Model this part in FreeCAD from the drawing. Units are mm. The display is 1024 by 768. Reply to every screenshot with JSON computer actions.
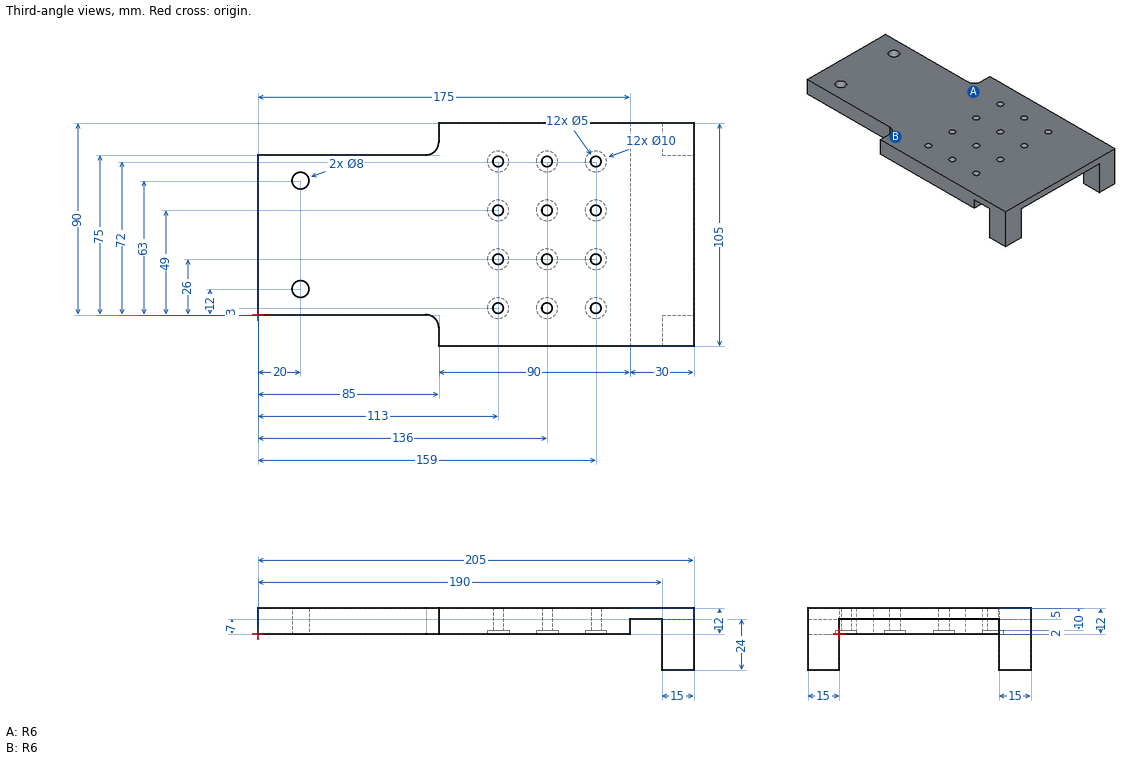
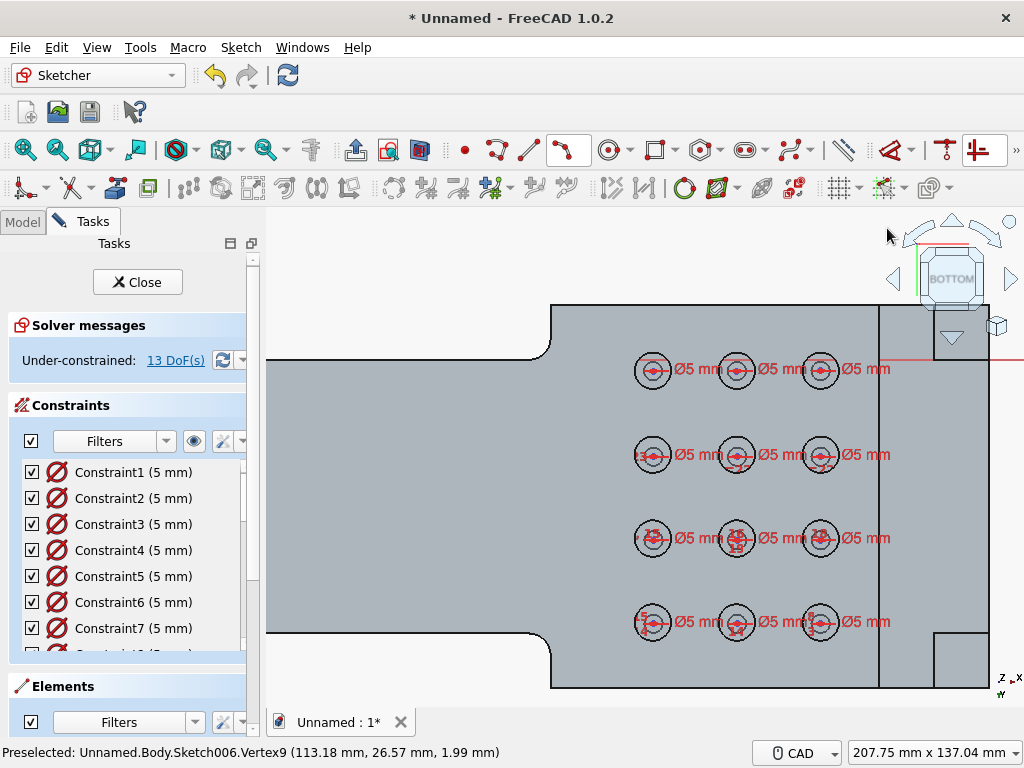
{"action": "left_click", "coordinate": [737, 457]}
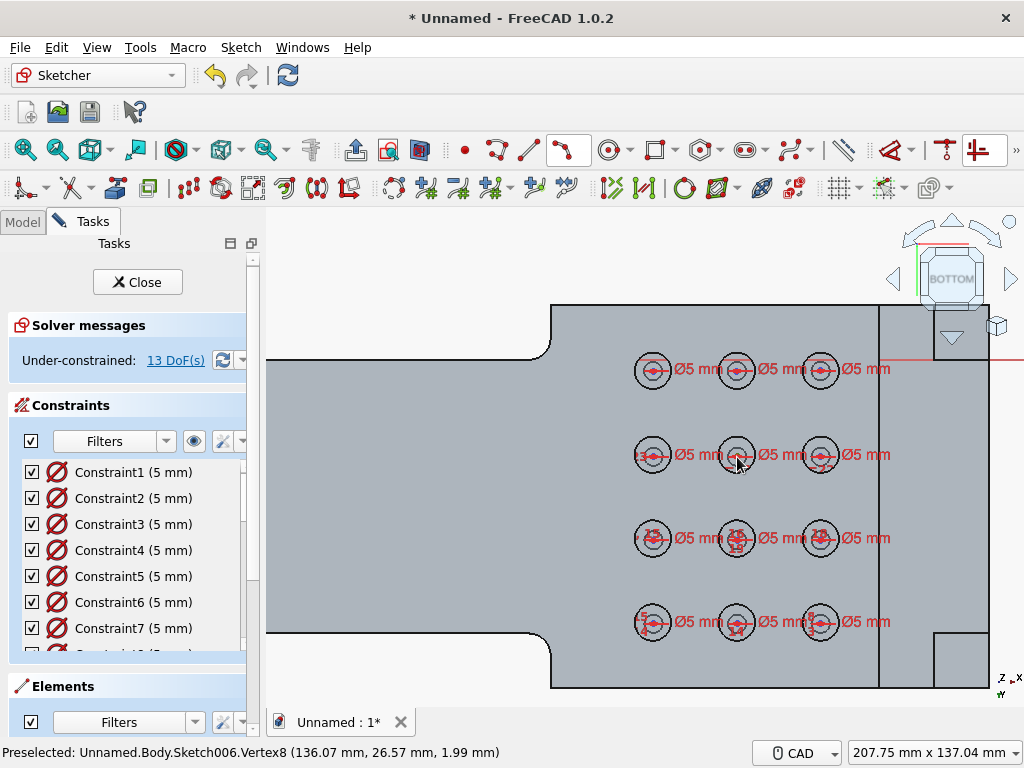
{"action": "left_click", "coordinate": [654, 457]}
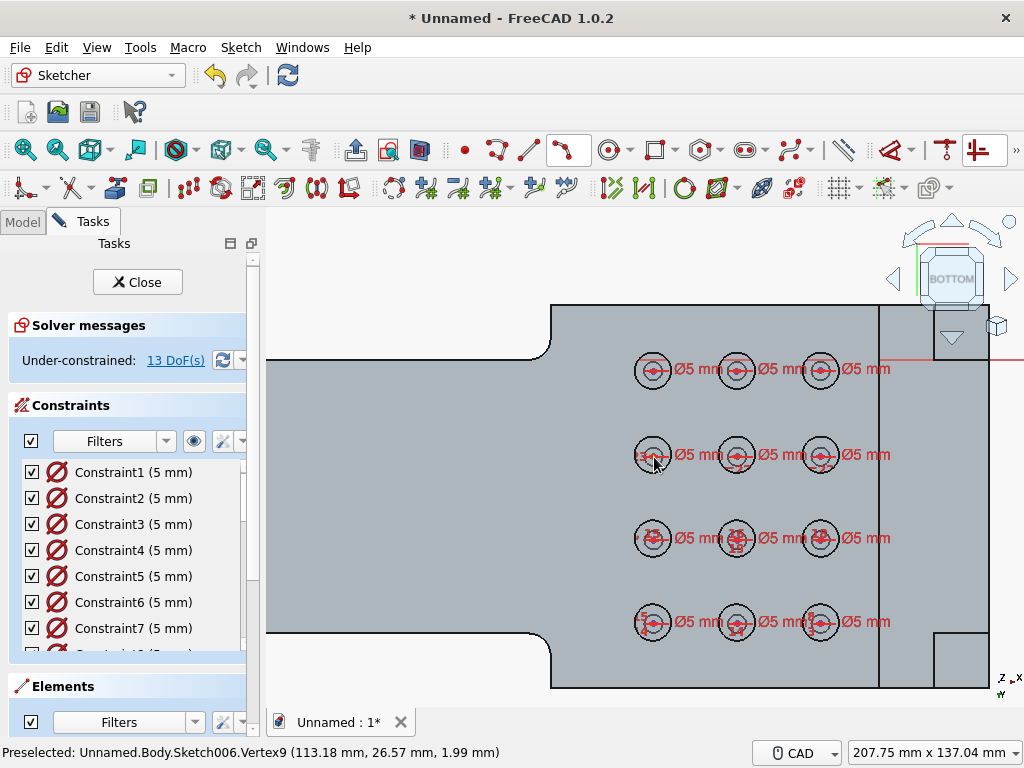
{"action": "key", "text": "h"}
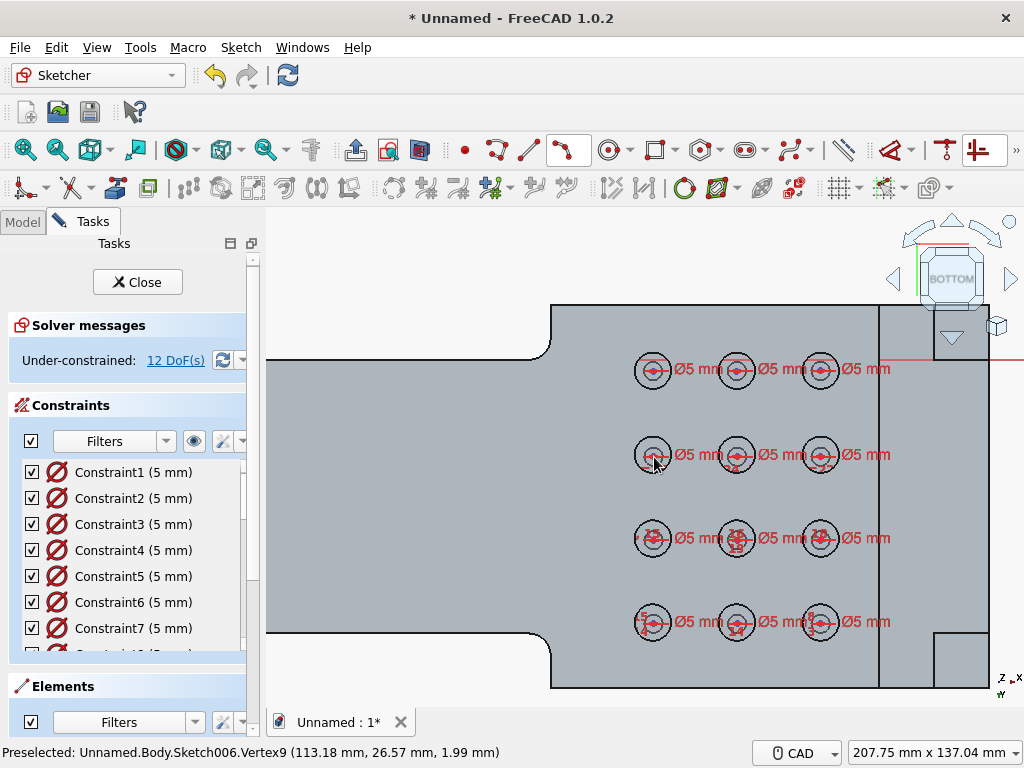
{"action": "left_click", "coordinate": [821, 457]}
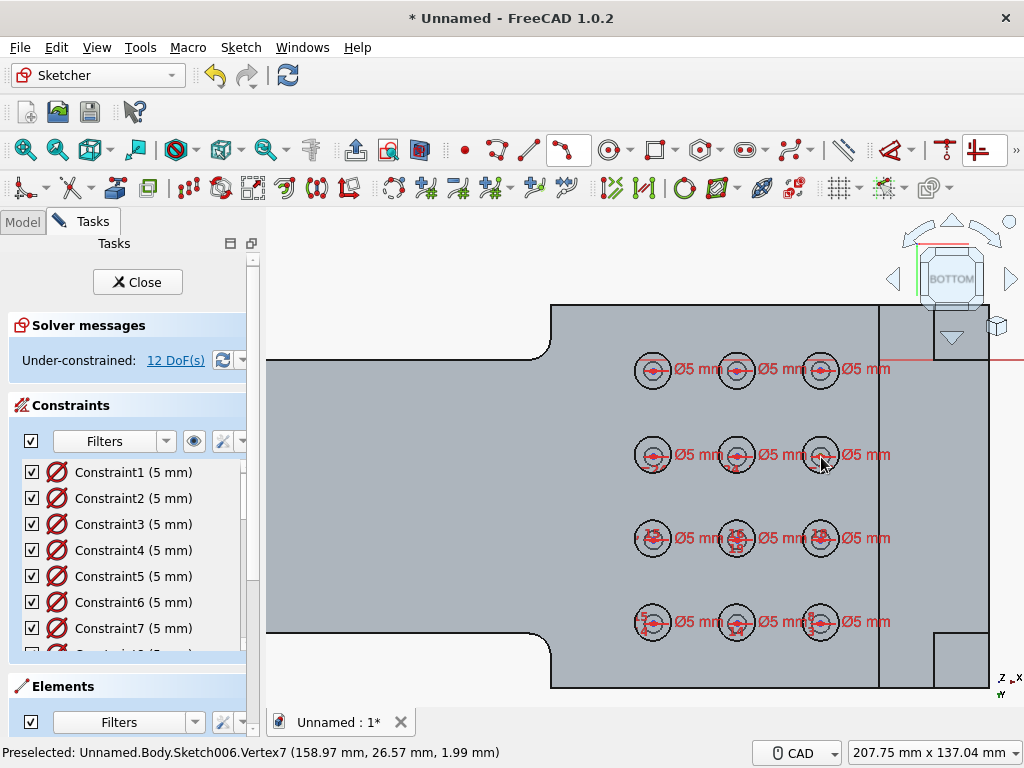
{"action": "left_click", "coordinate": [821, 371]}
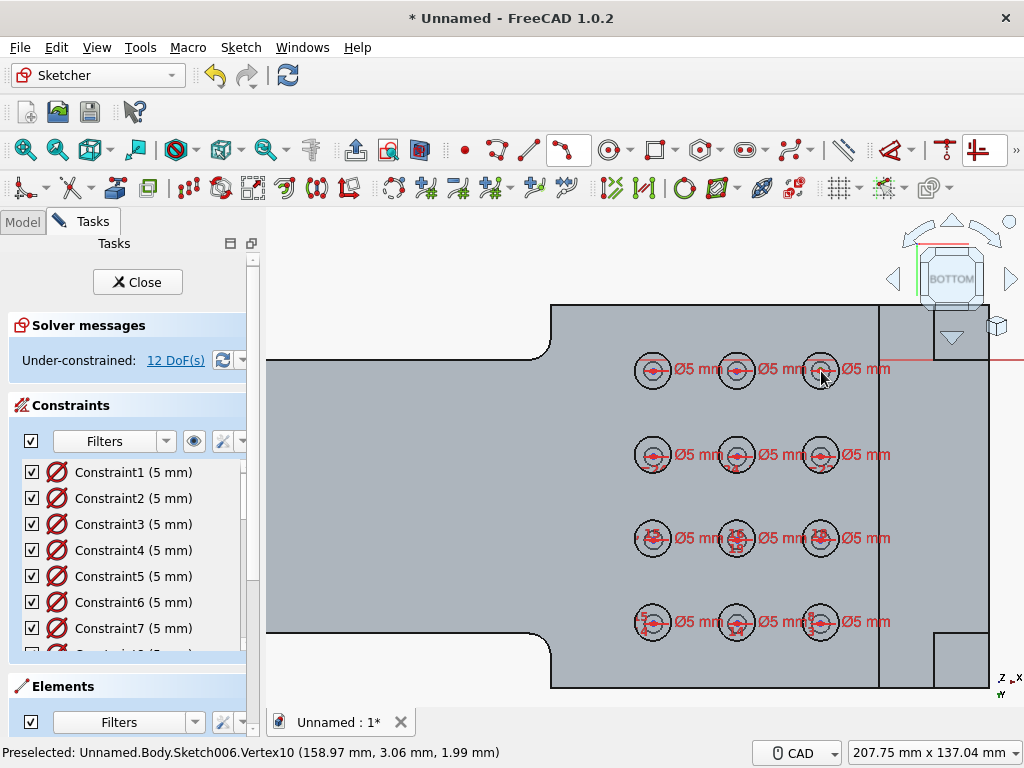
{"action": "left_click", "coordinate": [1002, 150]}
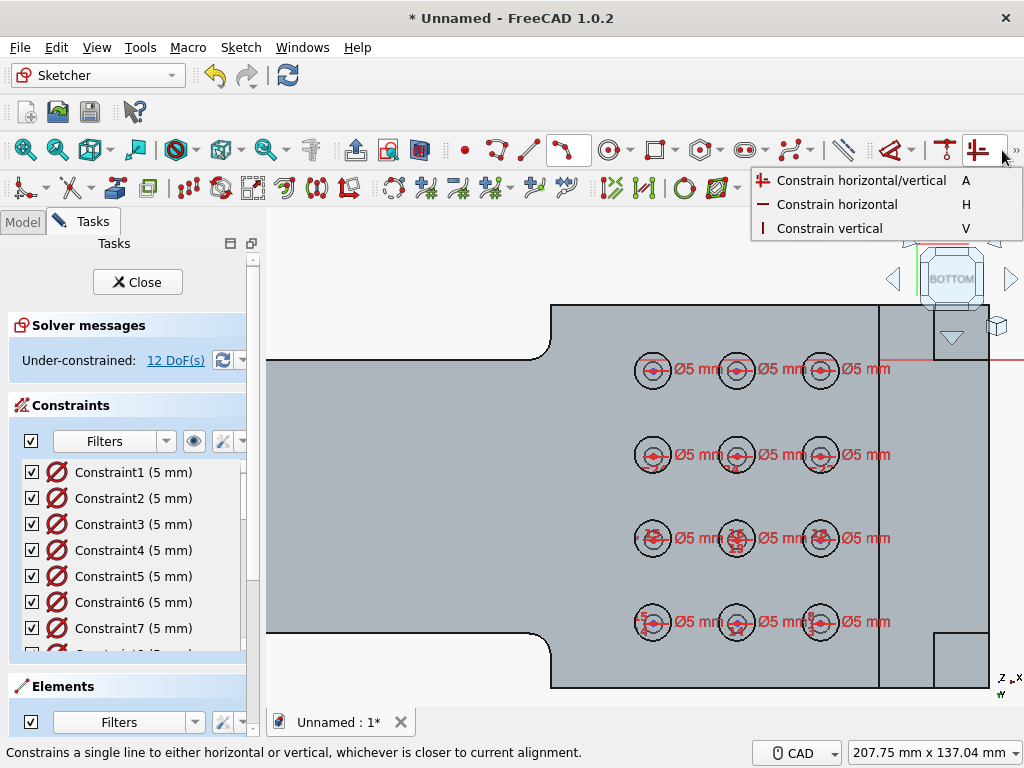
{"action": "left_click", "coordinate": [887, 228]}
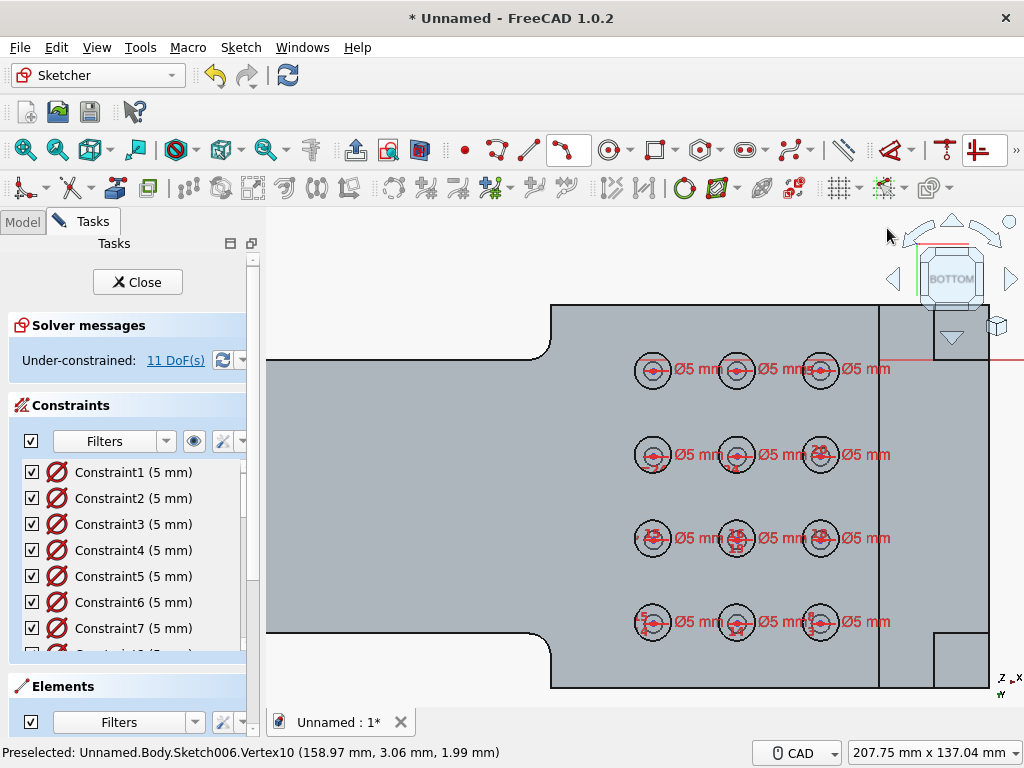
{"action": "left_click", "coordinate": [737, 457]}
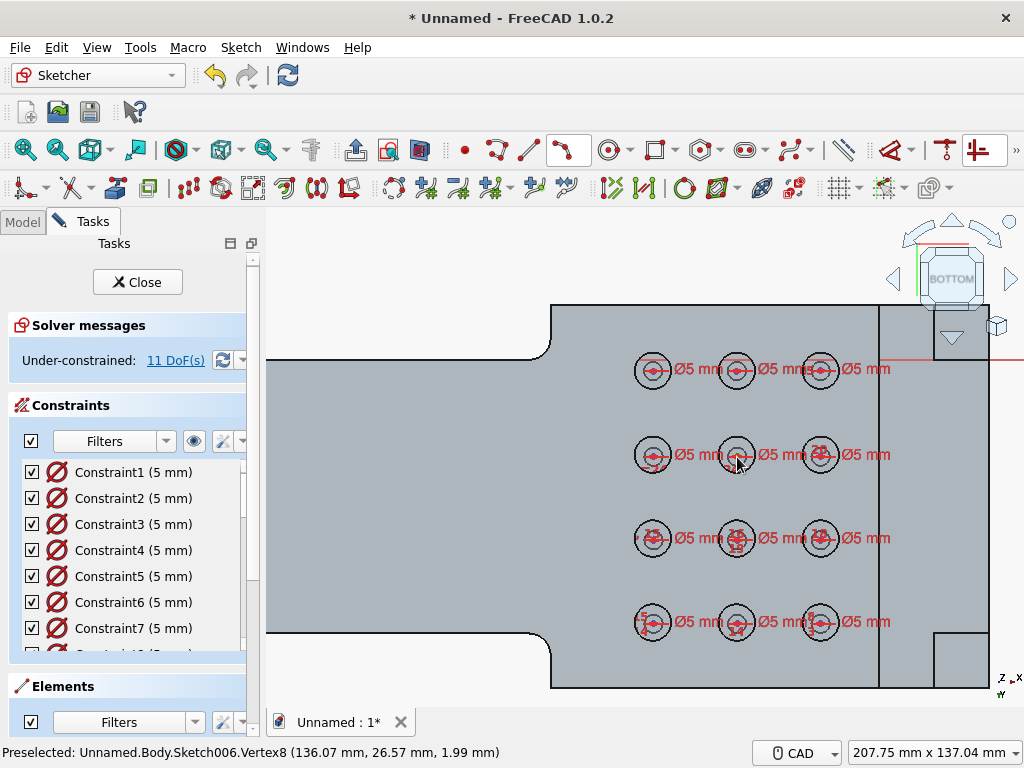
{"action": "left_click", "coordinate": [737, 371]}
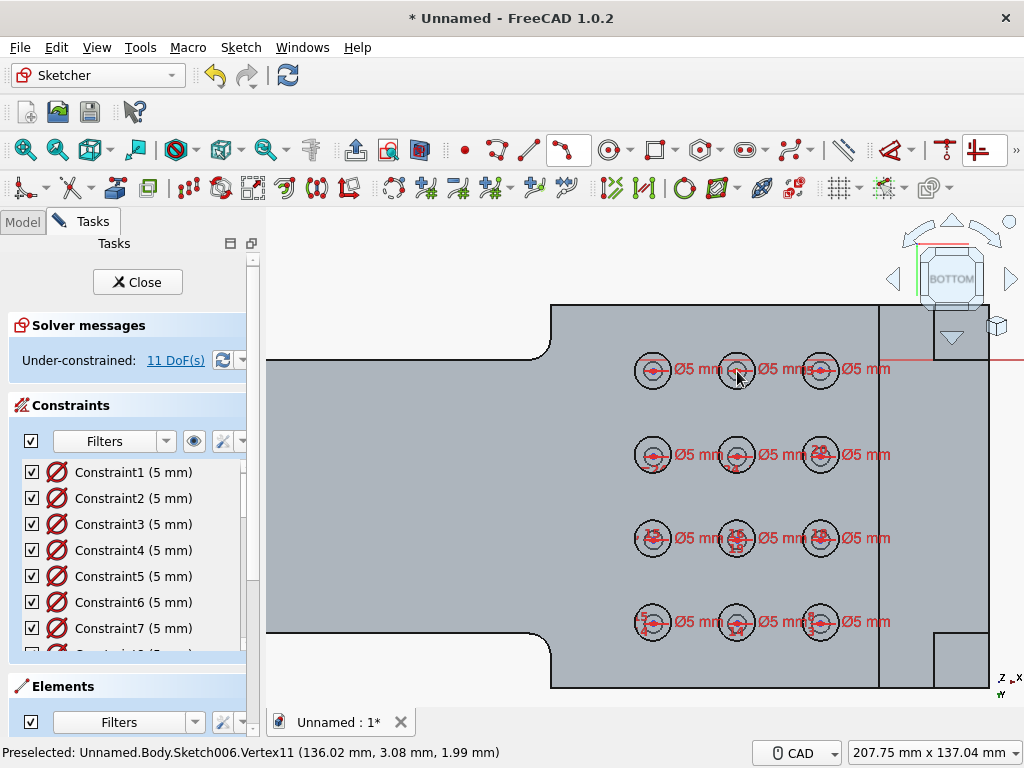
{"action": "key", "text": "v"}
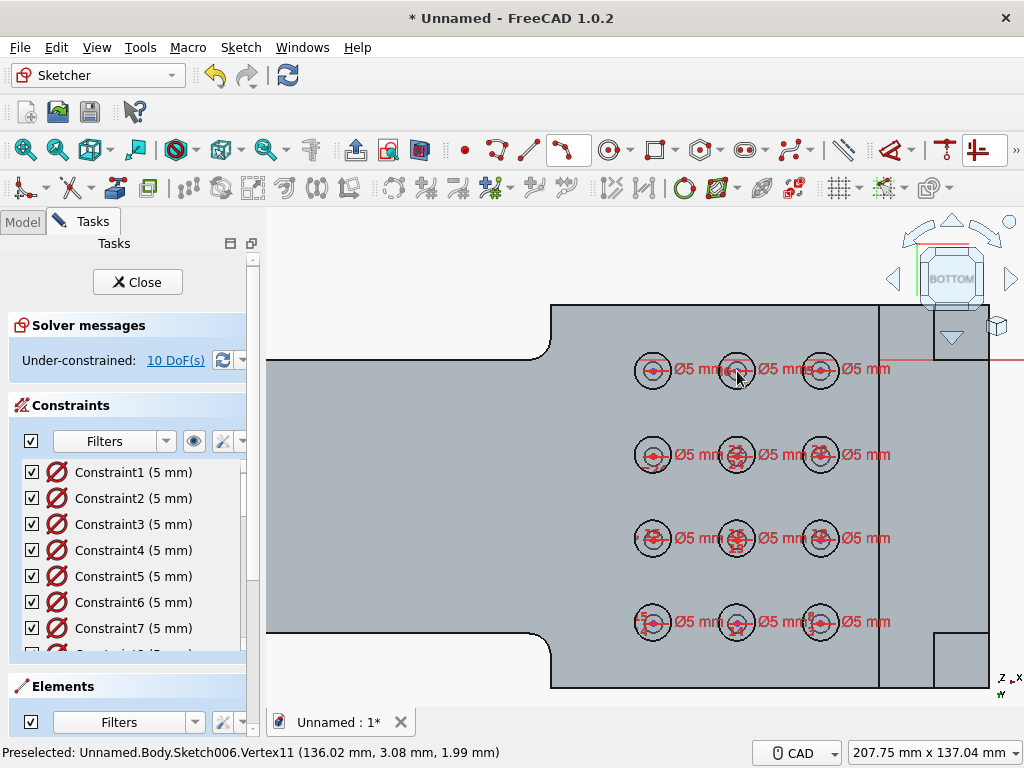
{"action": "left_click", "coordinate": [821, 371]}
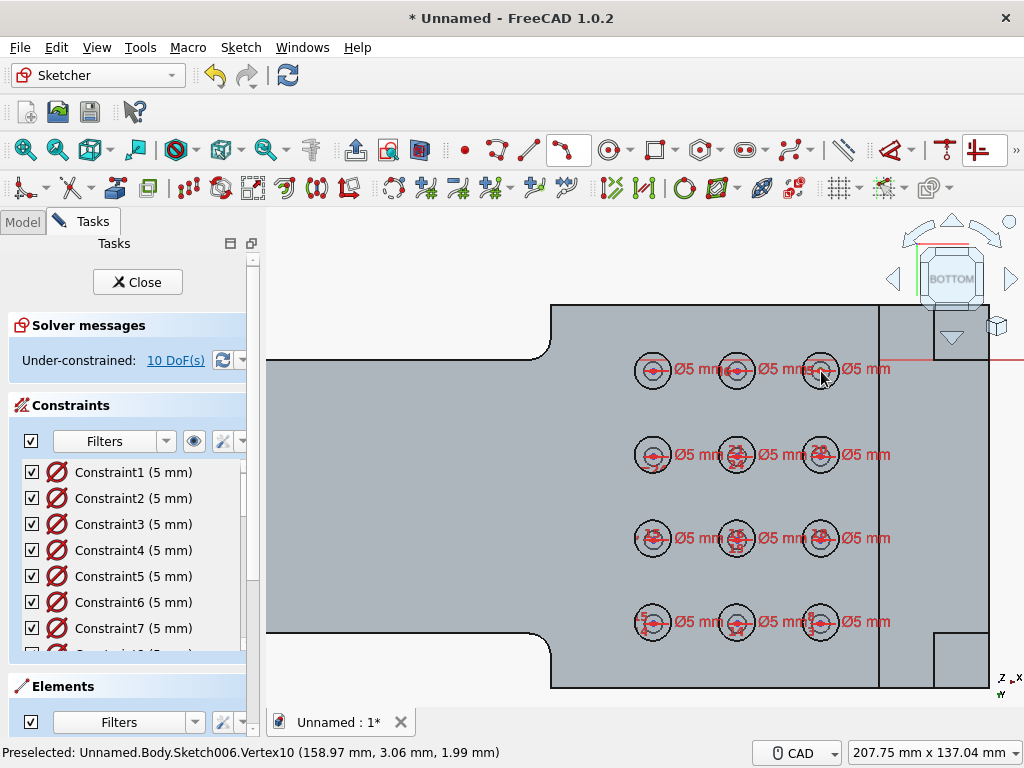
{"action": "left_click", "coordinate": [737, 371]}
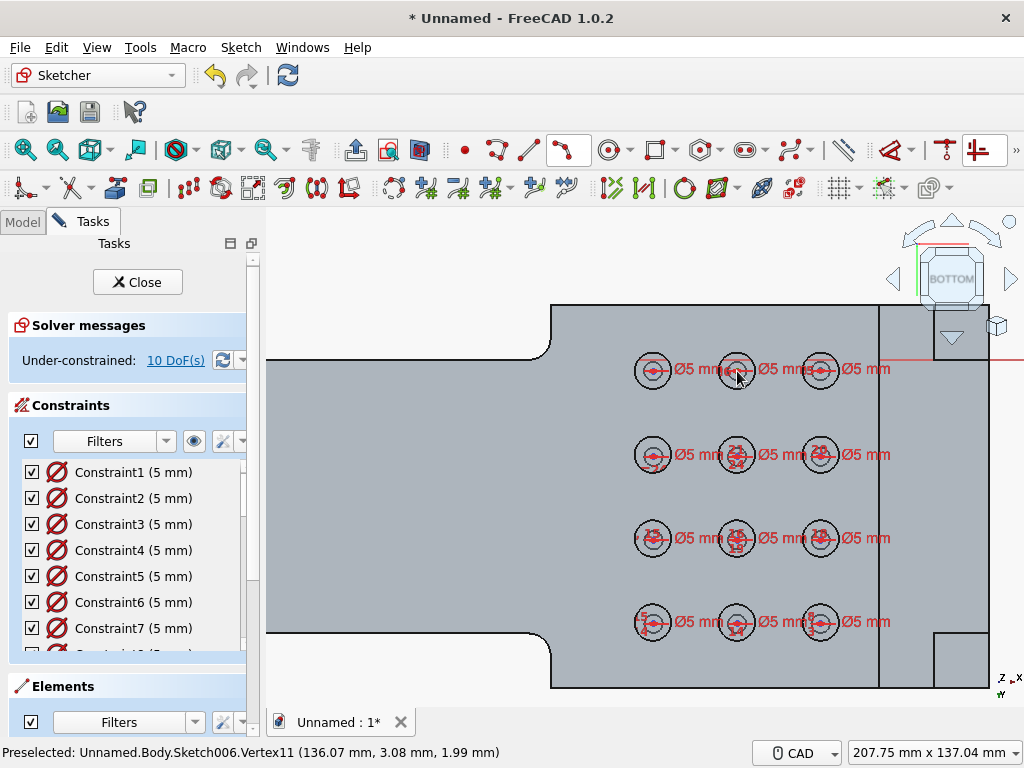
{"action": "key", "text": "h"}